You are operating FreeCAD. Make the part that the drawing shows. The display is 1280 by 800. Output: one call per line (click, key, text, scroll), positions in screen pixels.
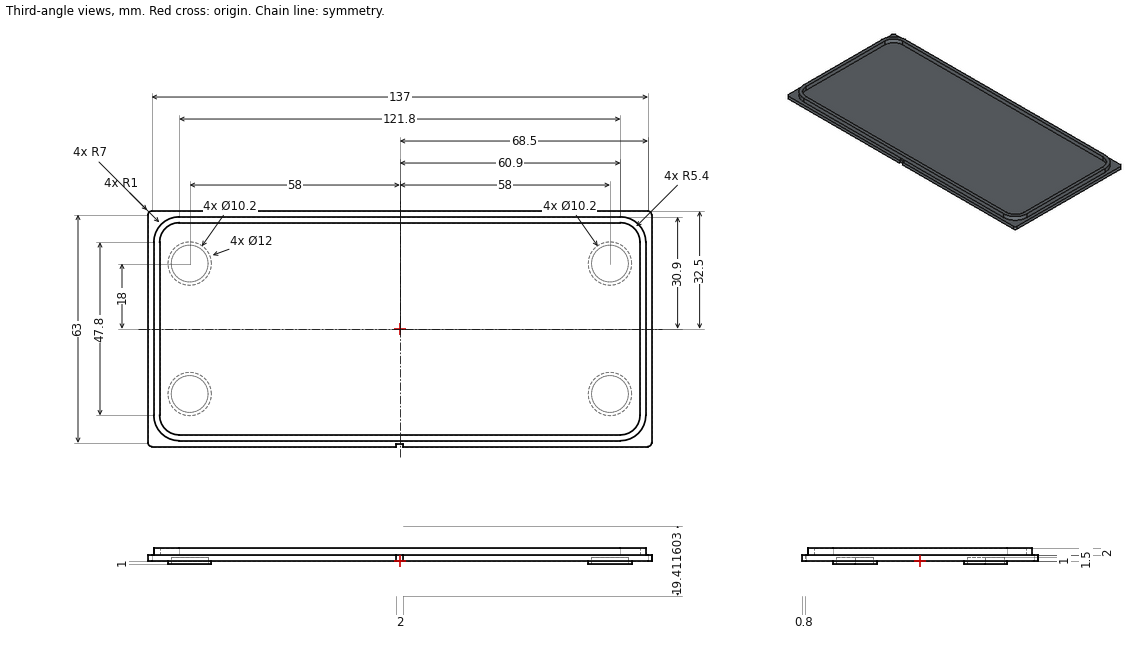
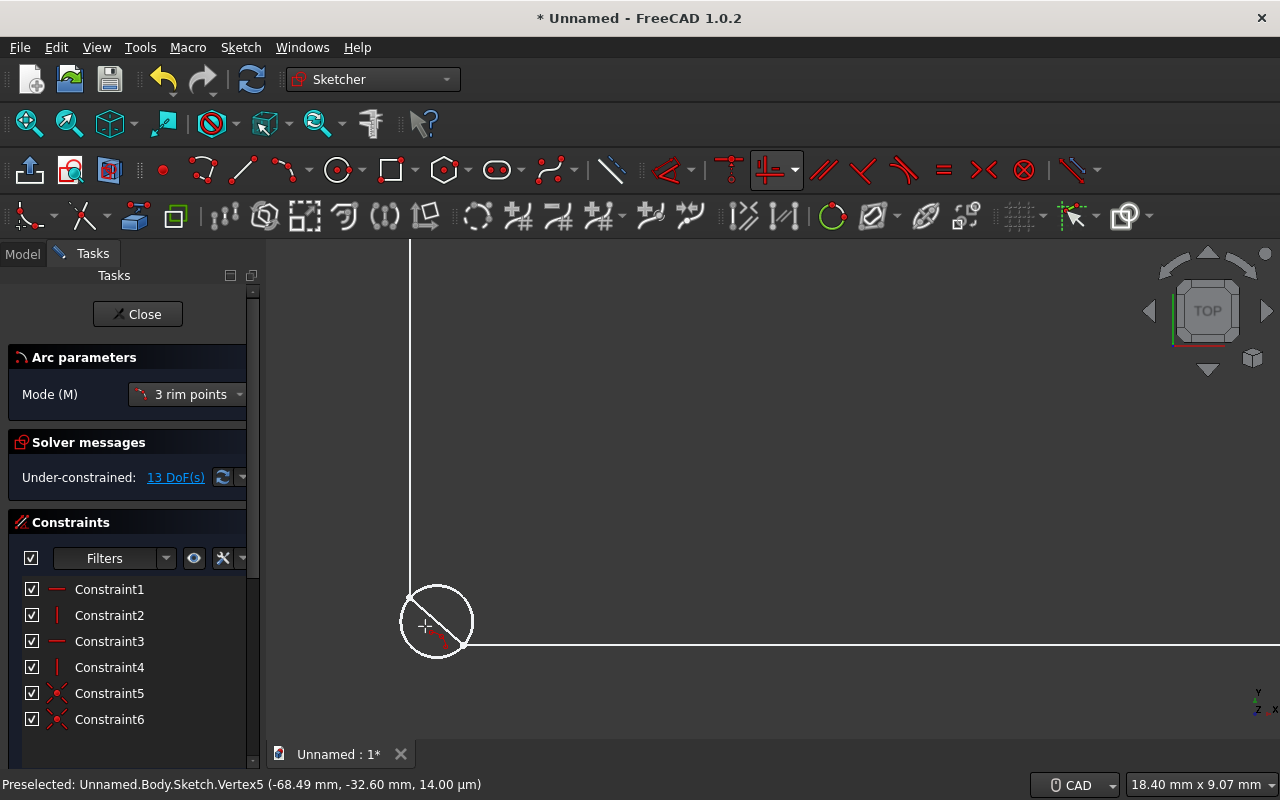
click(425, 624)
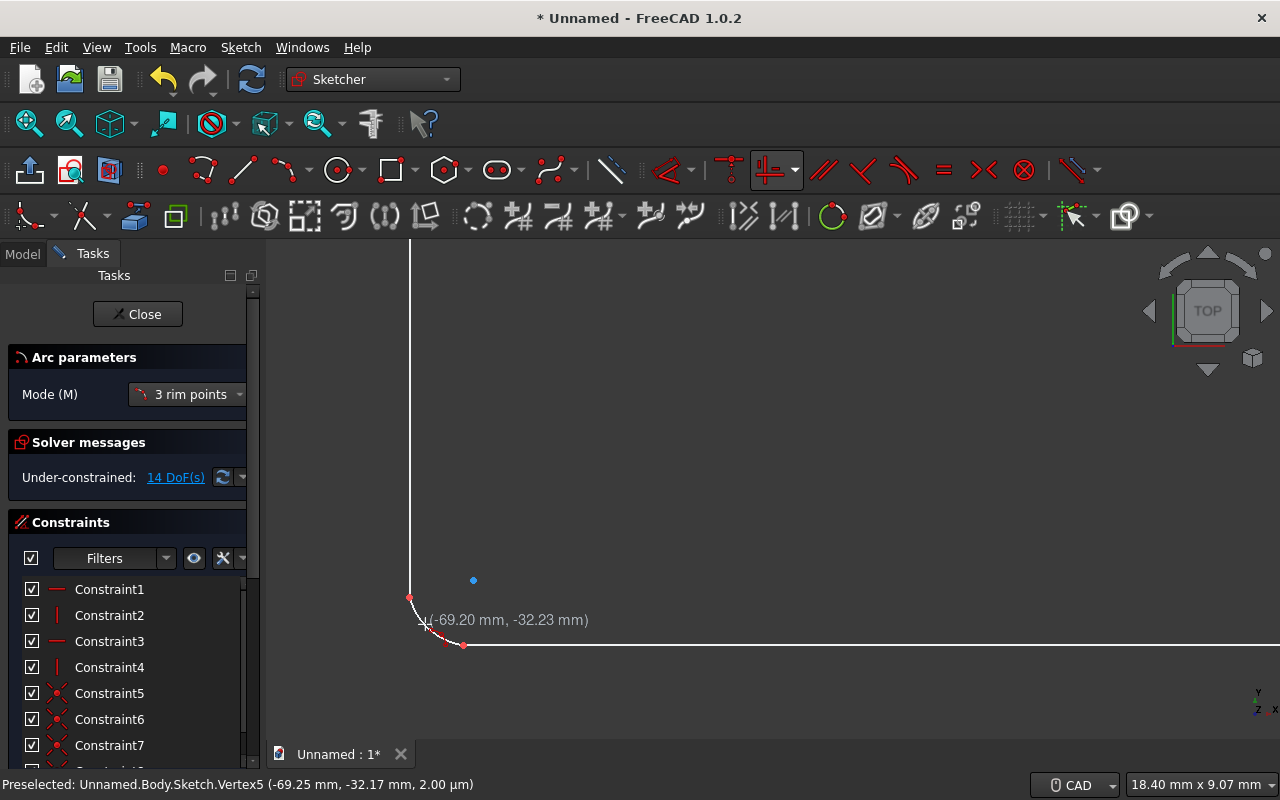
scroll(421, 621, down, 13)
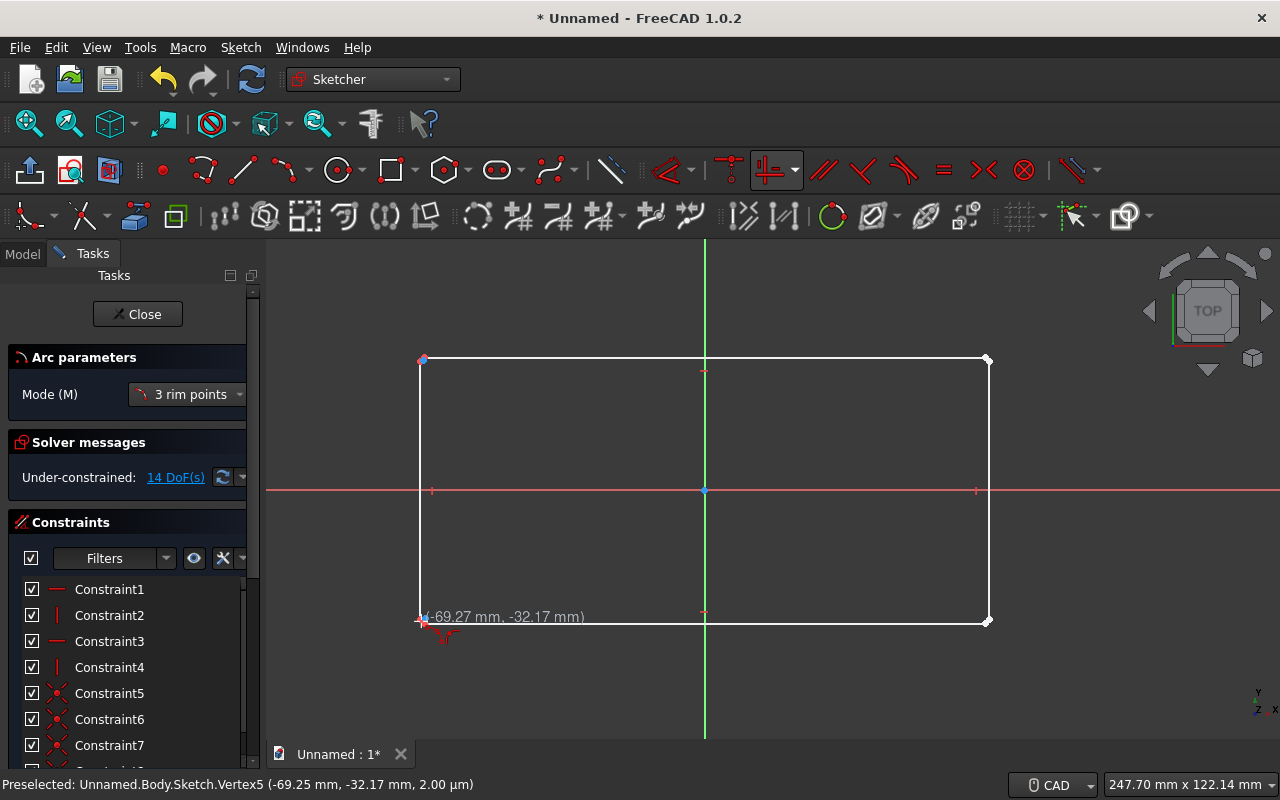
scroll(985, 623, up, 6)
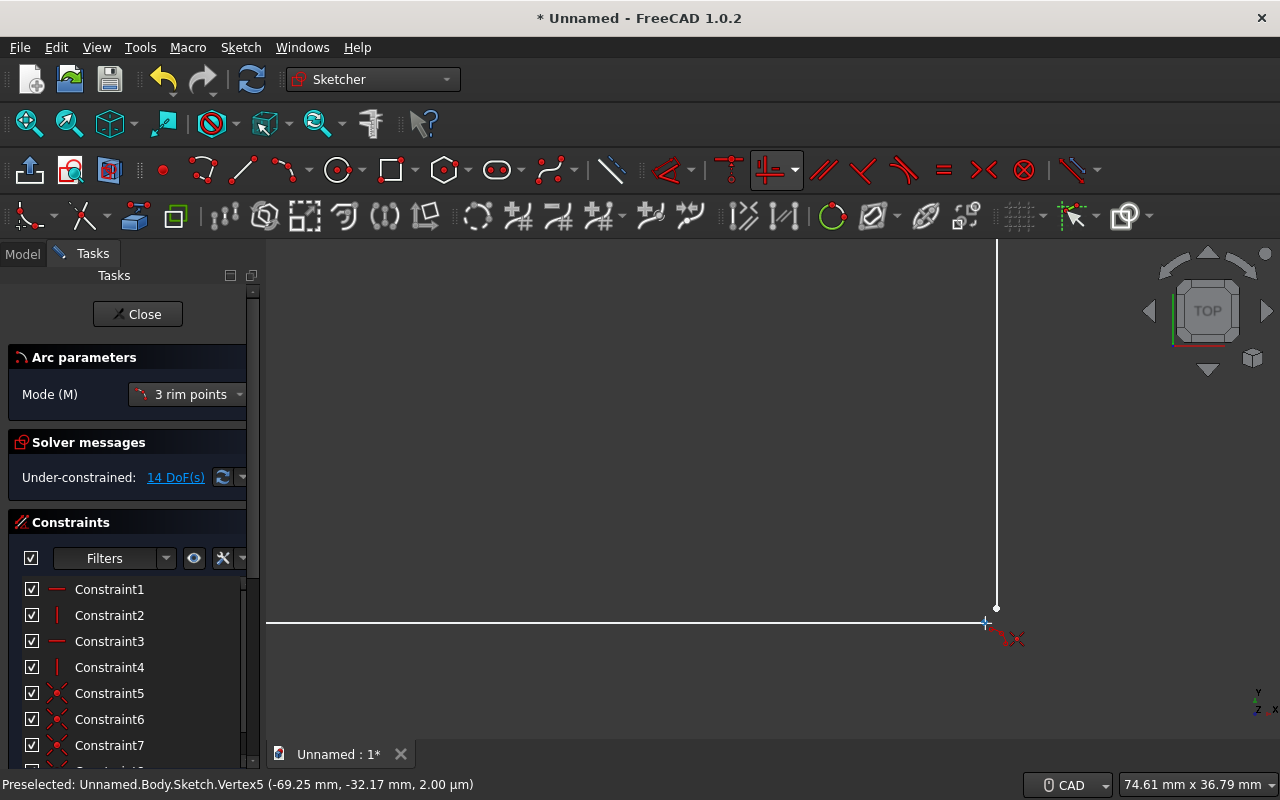
click(984, 623)
click(997, 609)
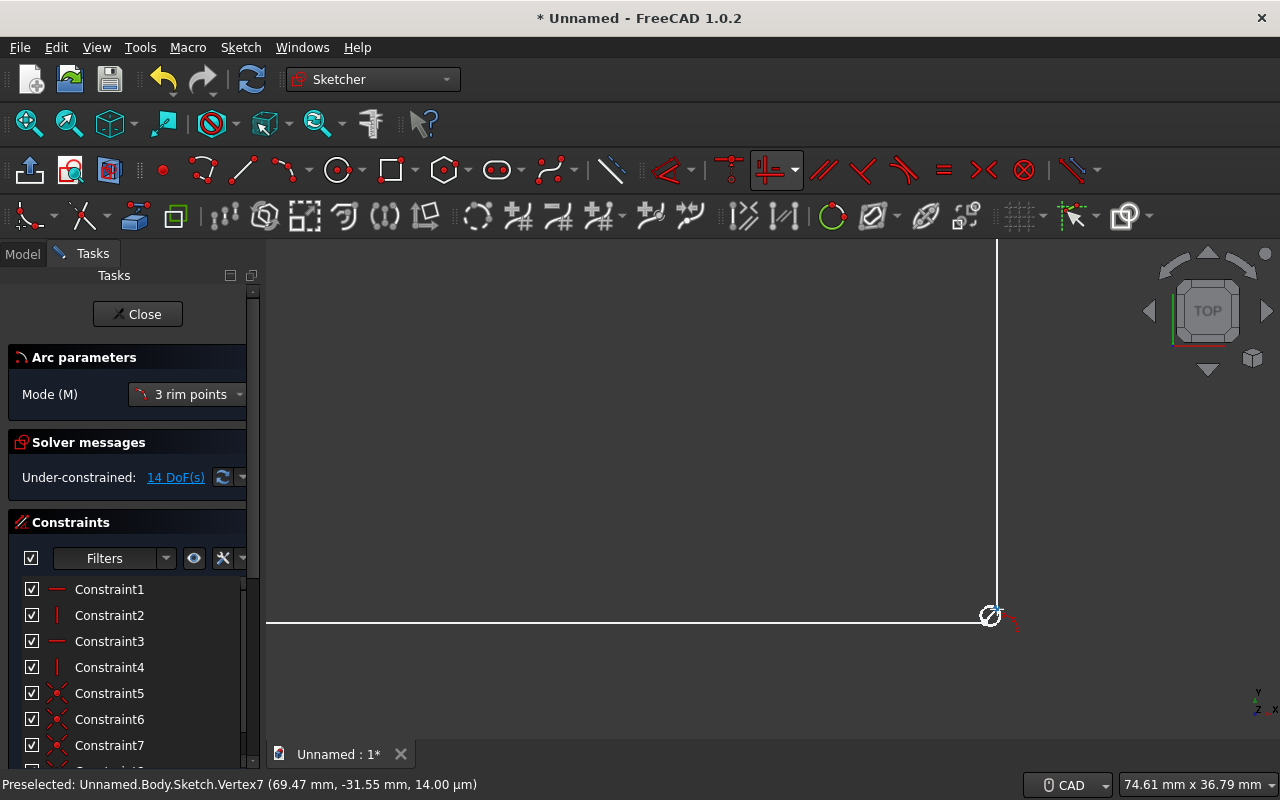
scroll(993, 618, up, 7)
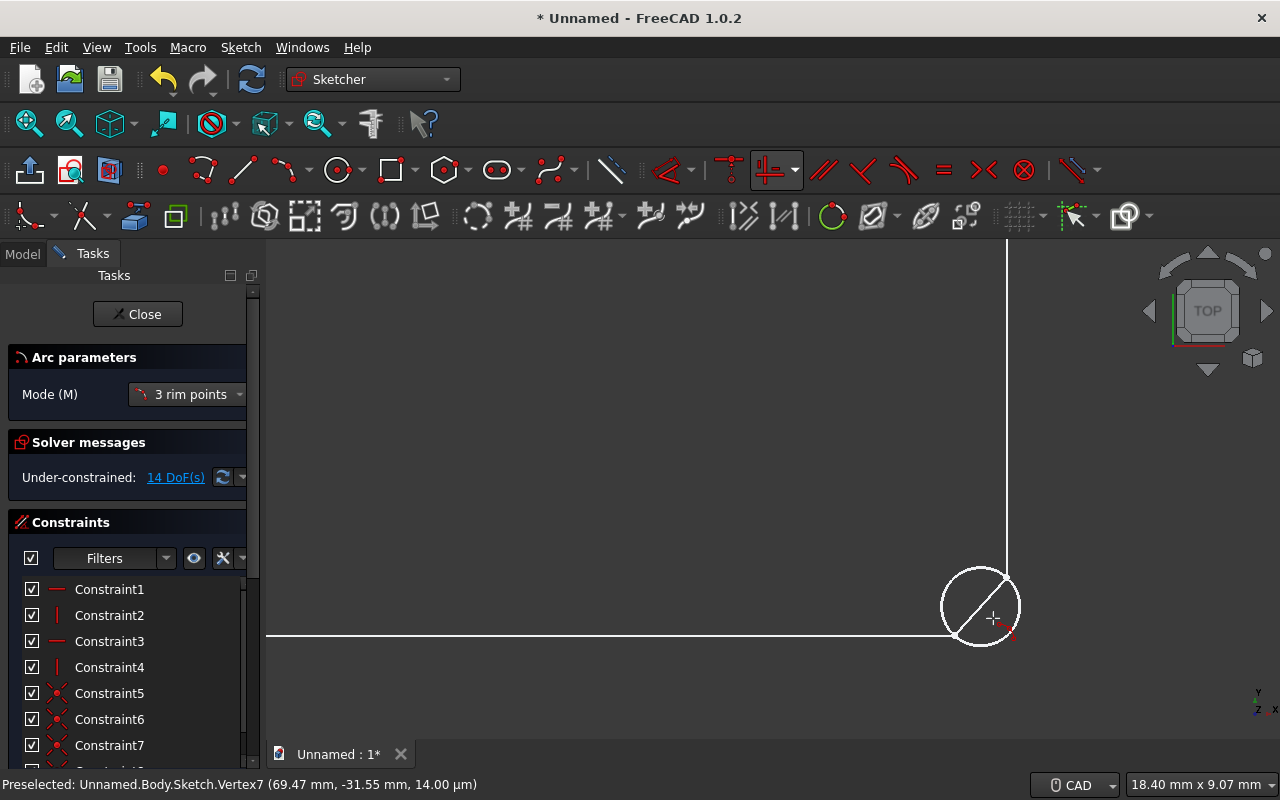
click(992, 614)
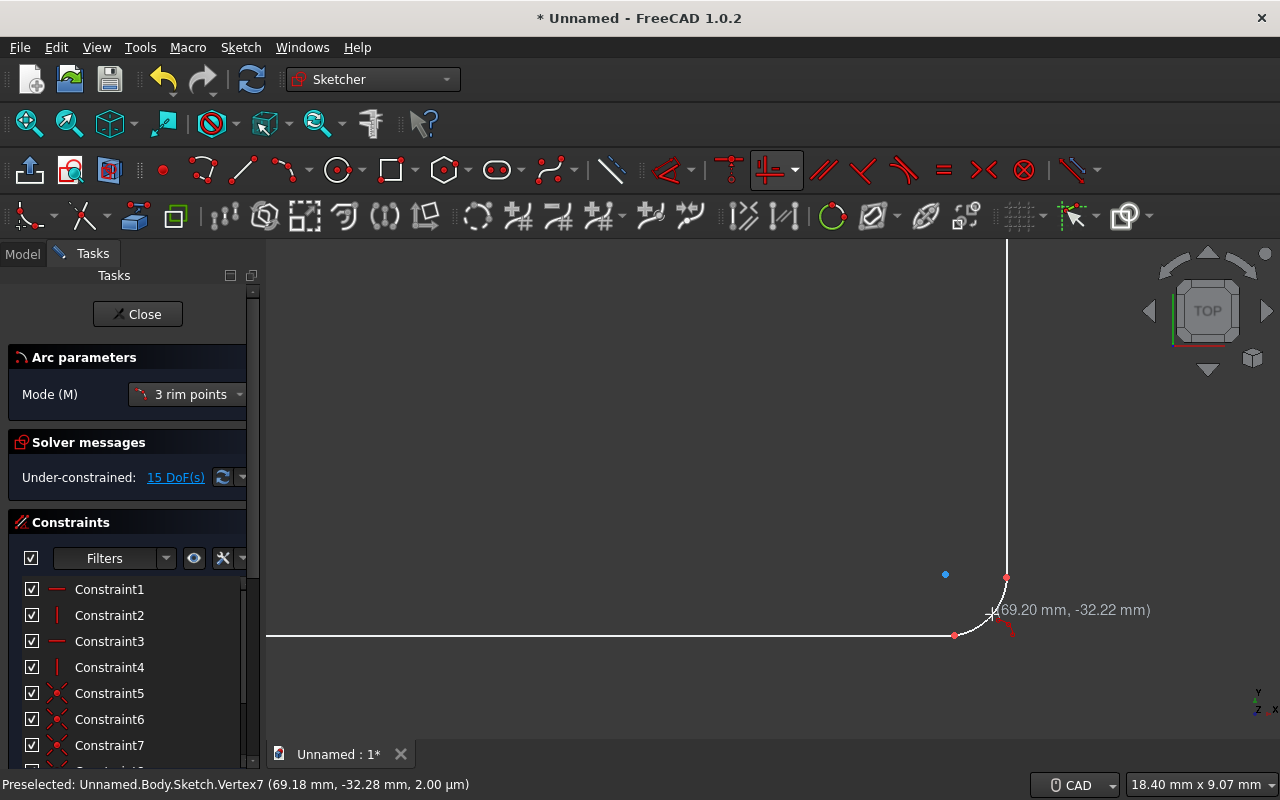
scroll(987, 621, down, 13)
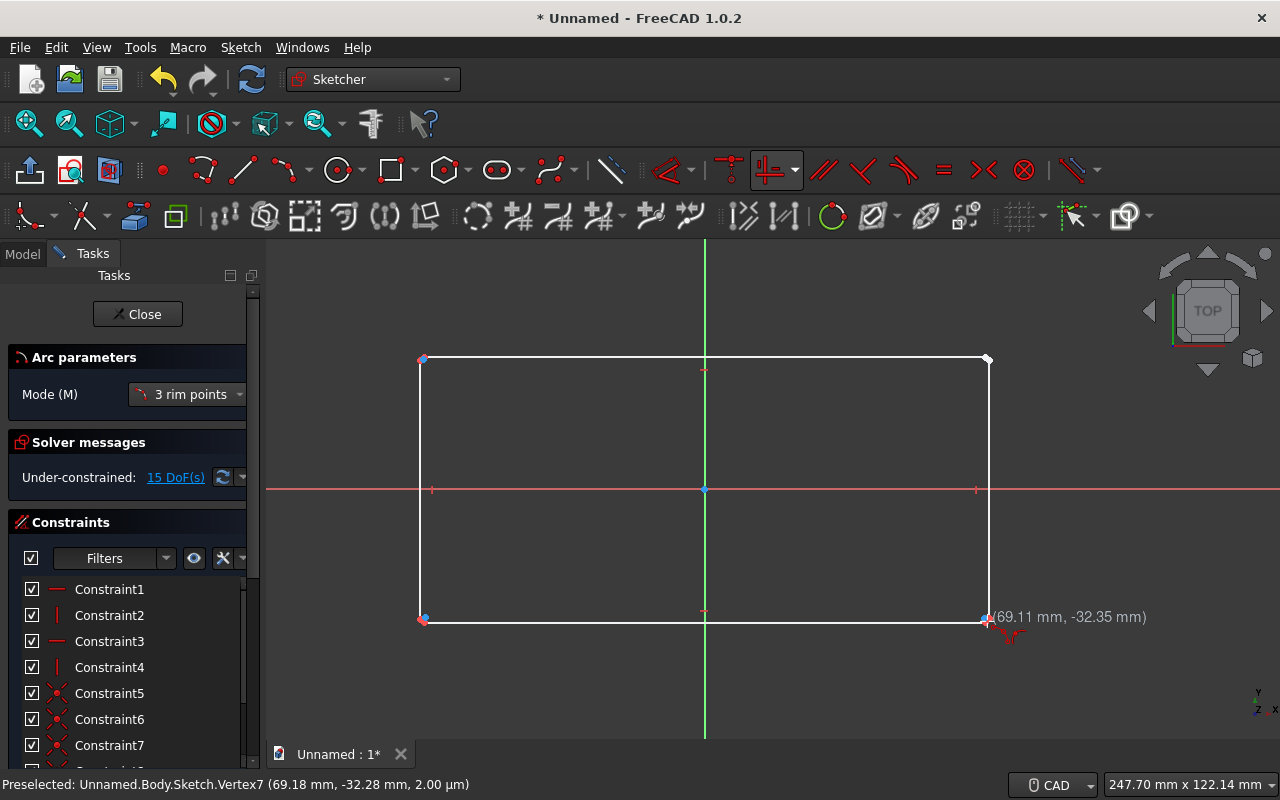
scroll(989, 360, up, 6)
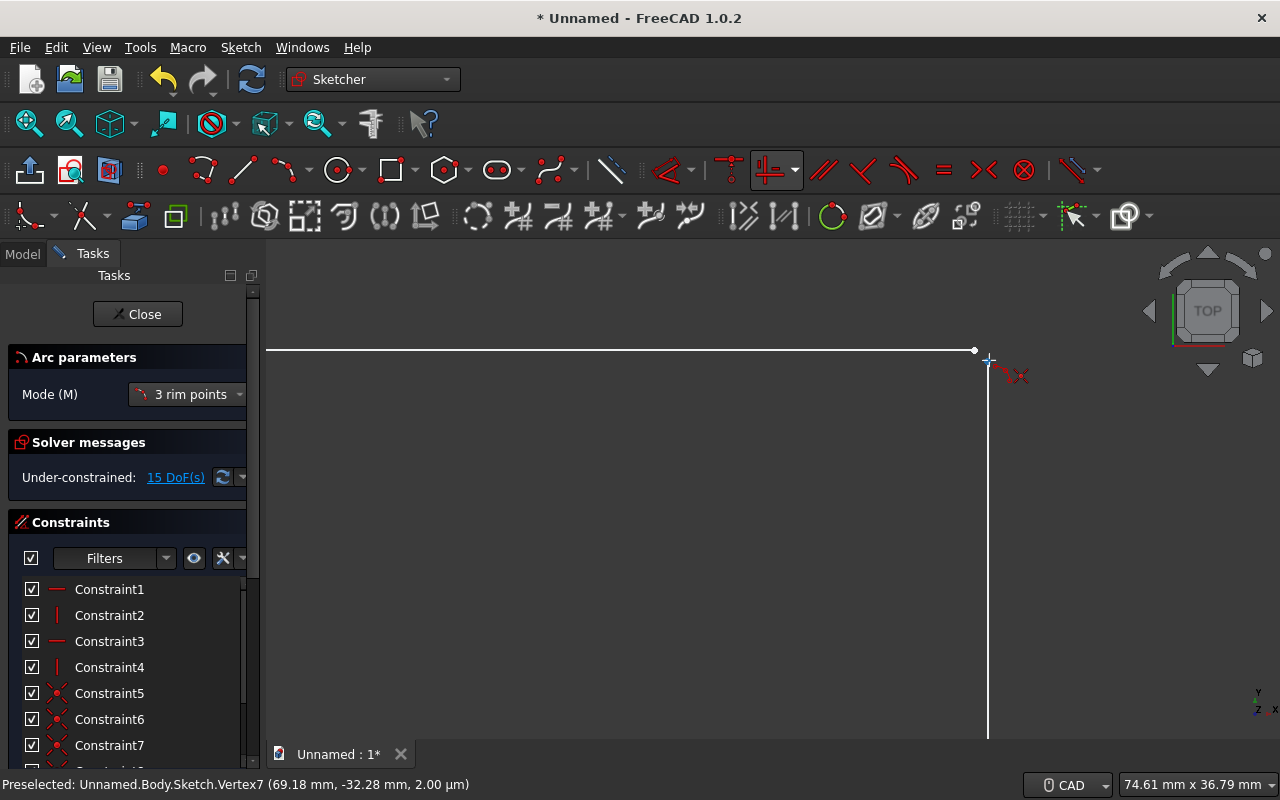
click(988, 362)
click(975, 350)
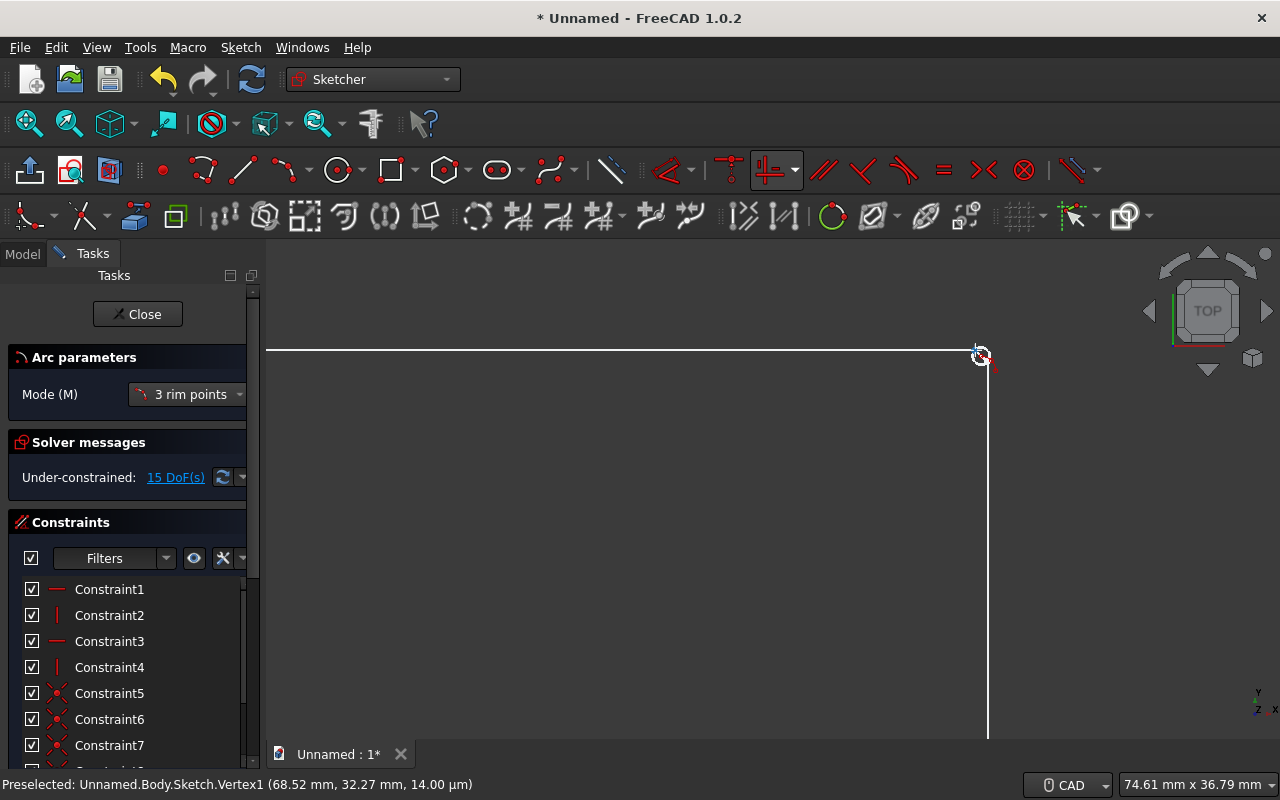
scroll(984, 351, up, 7)